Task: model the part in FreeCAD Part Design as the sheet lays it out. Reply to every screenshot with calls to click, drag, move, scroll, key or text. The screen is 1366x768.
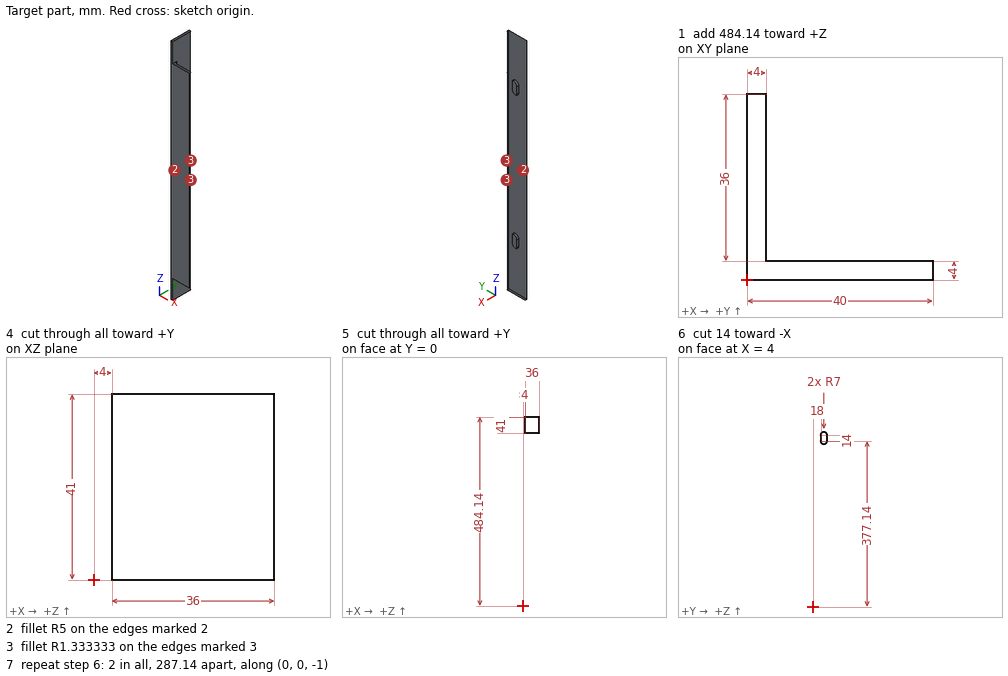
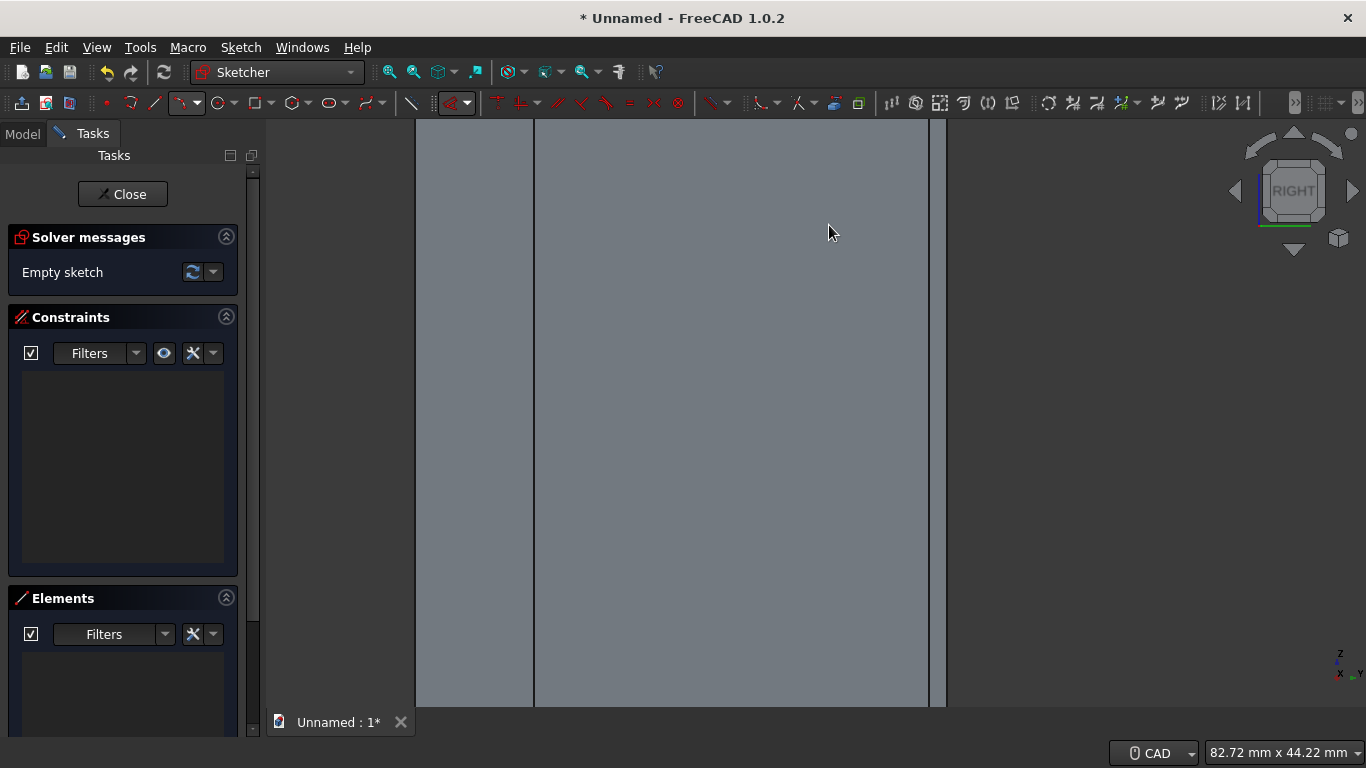
click(330, 104)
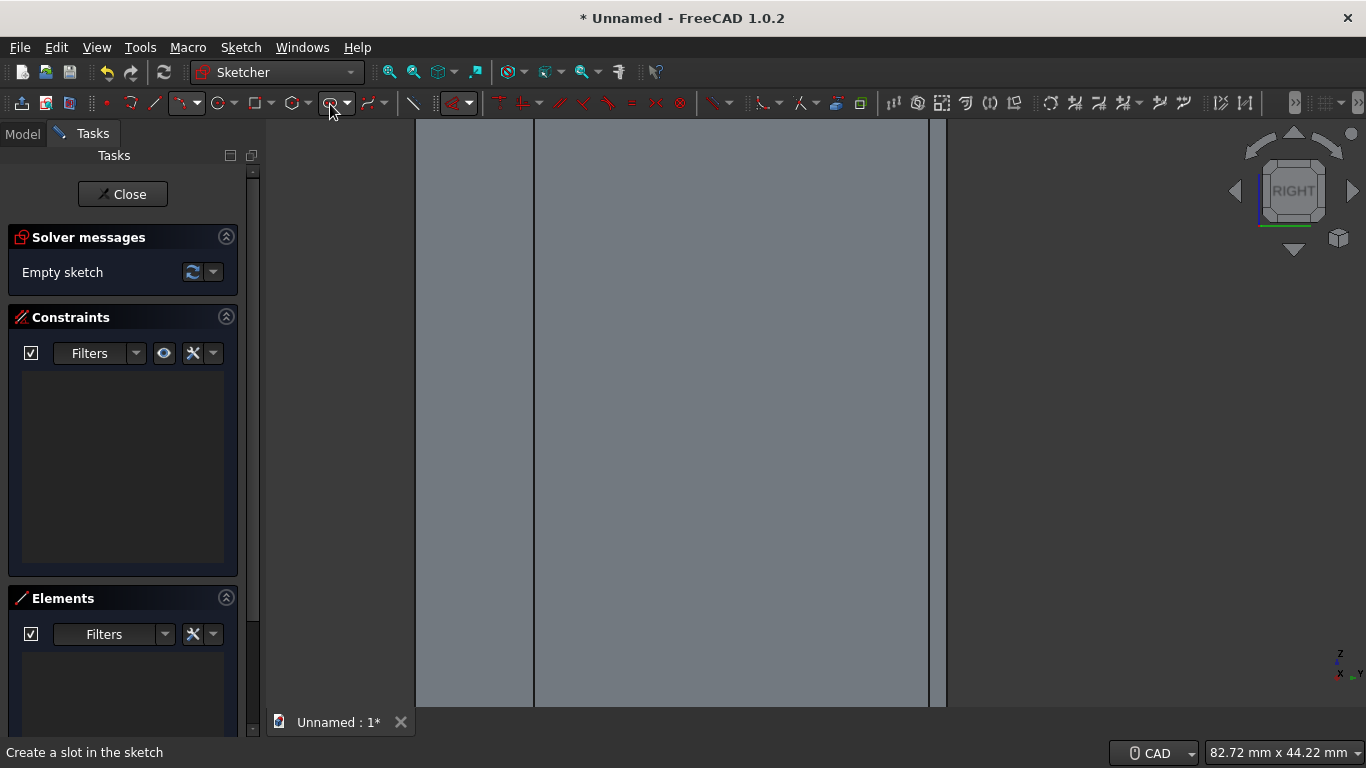
click(747, 499)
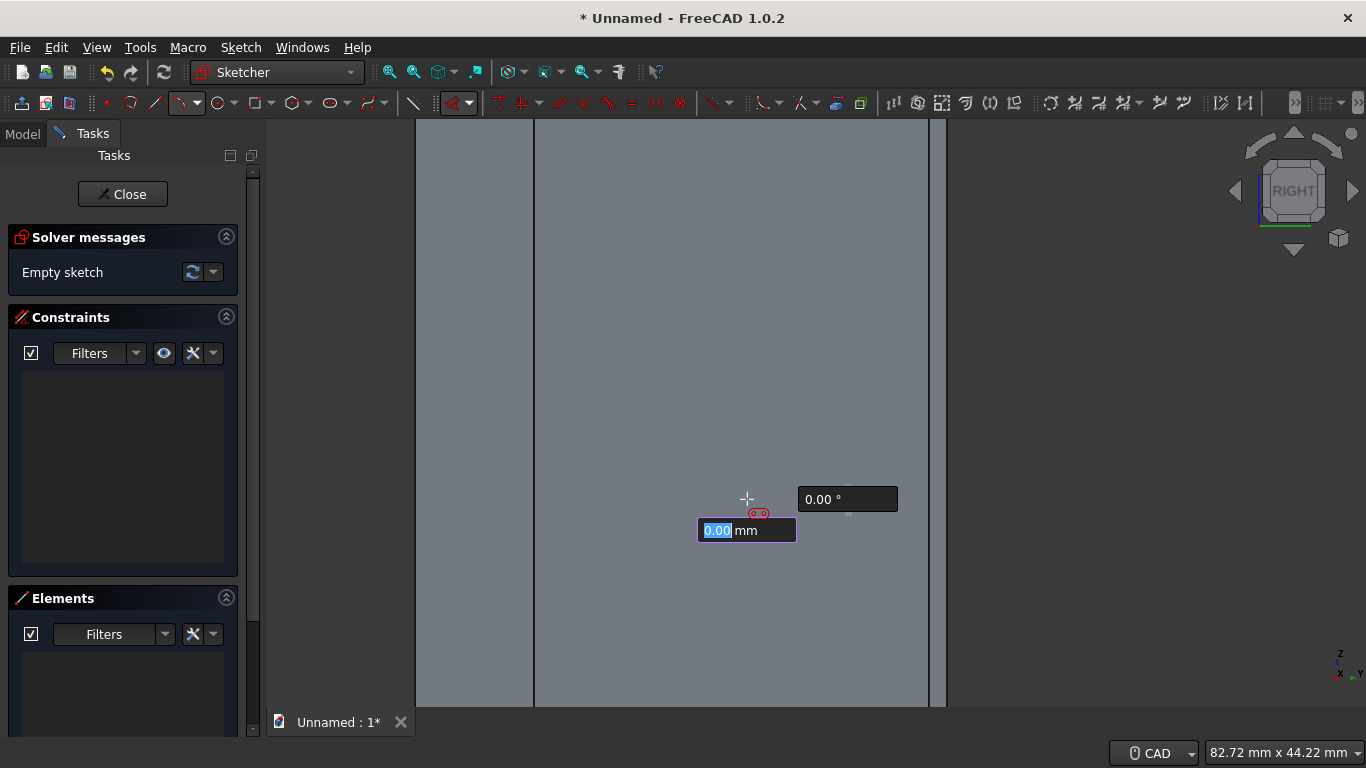
click(747, 313)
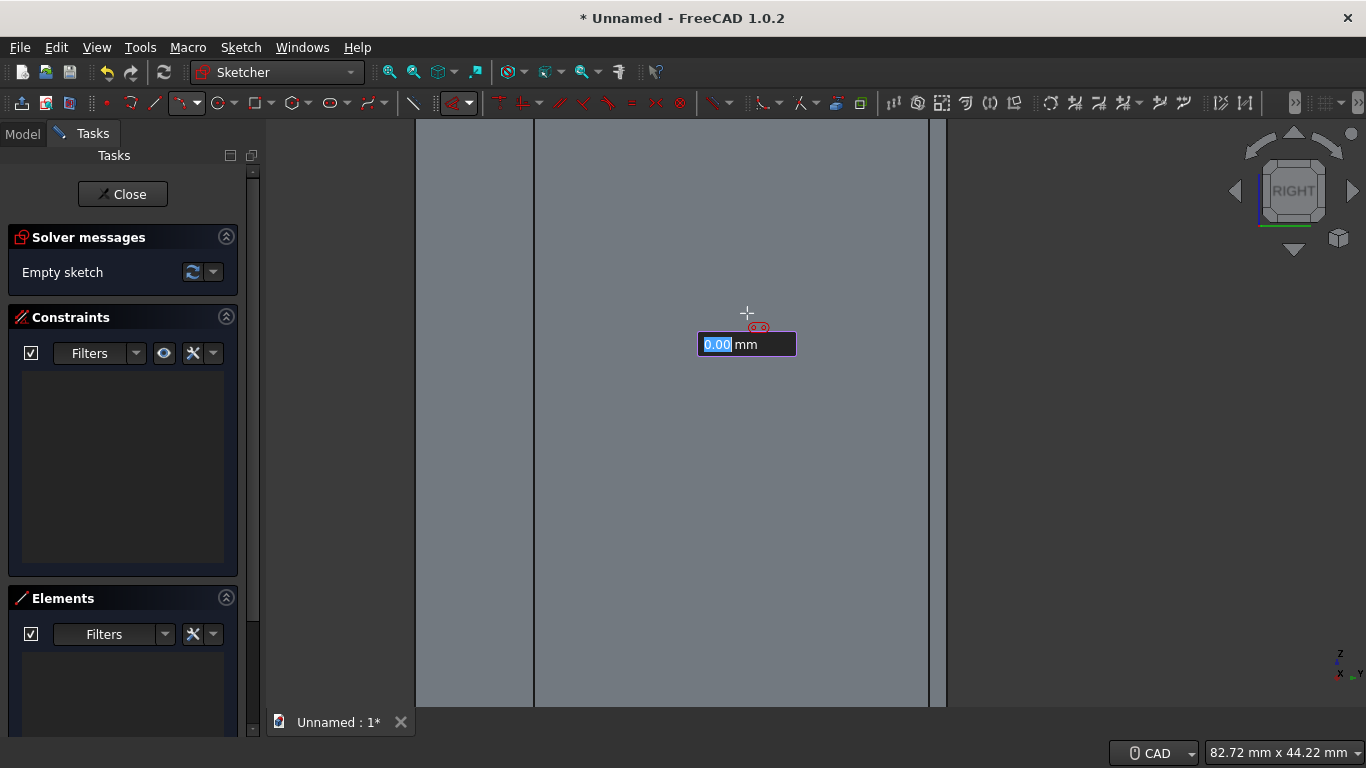
click(840, 406)
key(Escape)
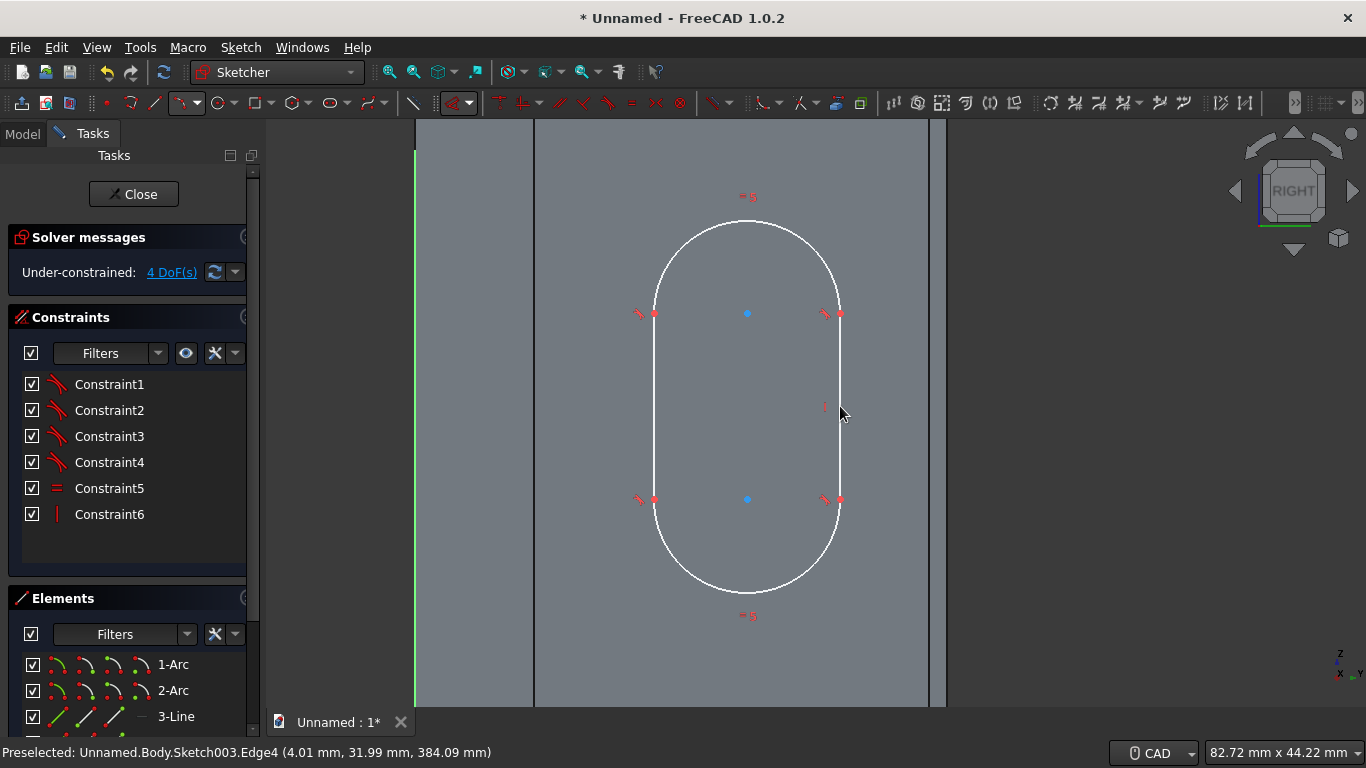
click(692, 575)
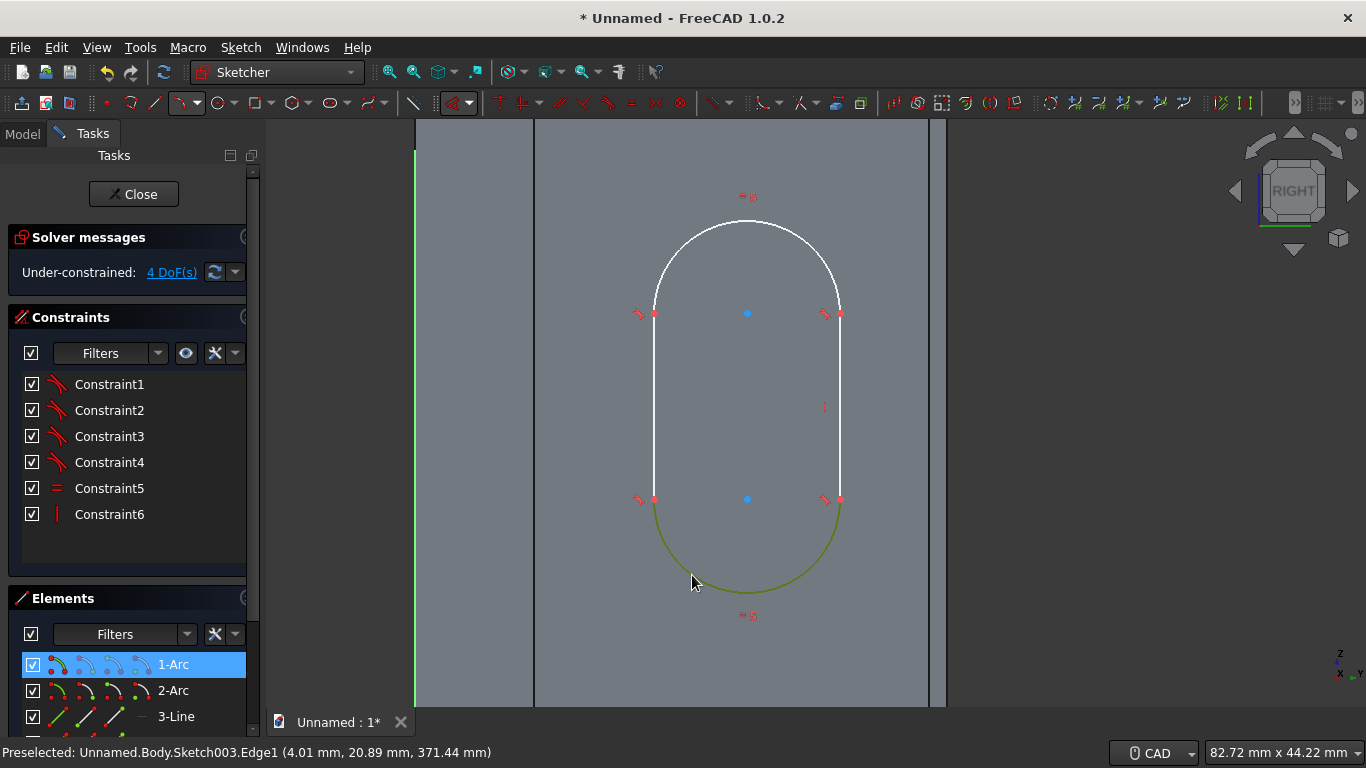
click(472, 104)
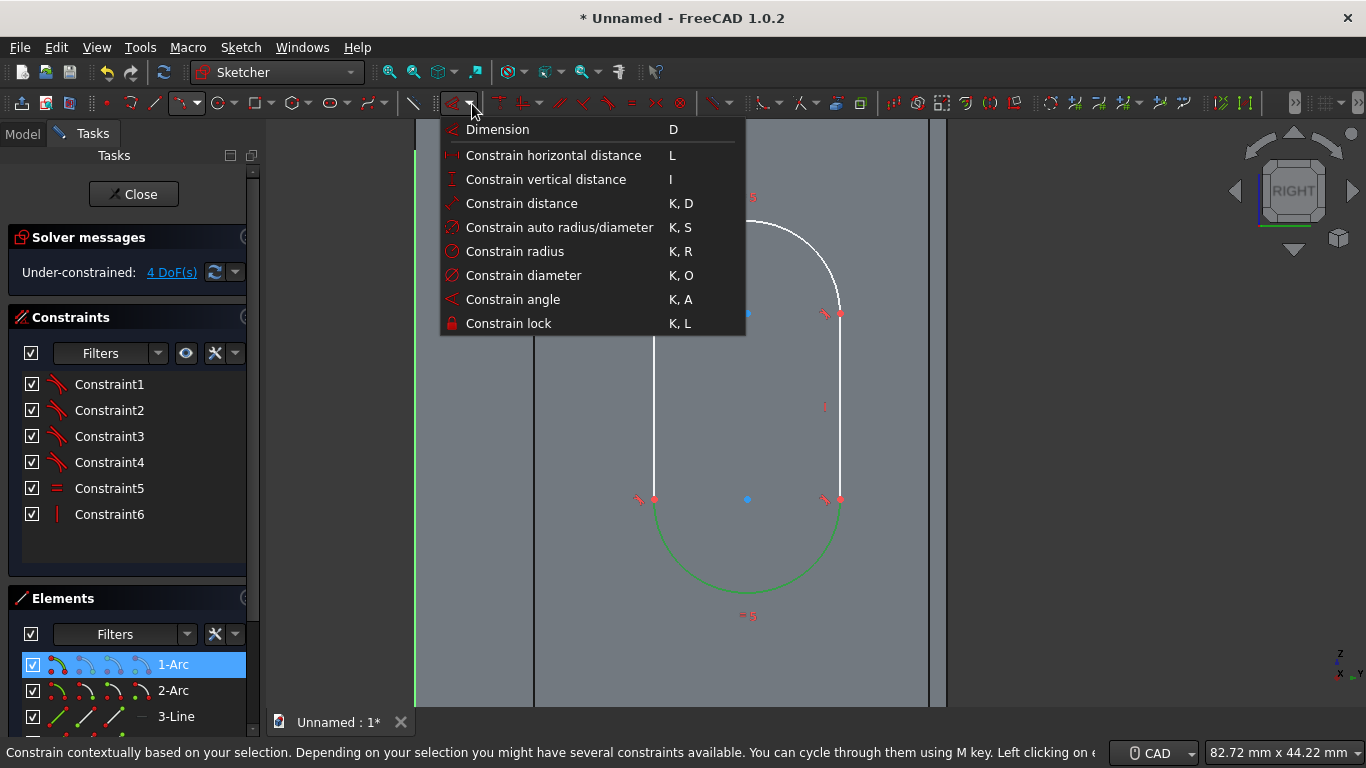
click(593, 251)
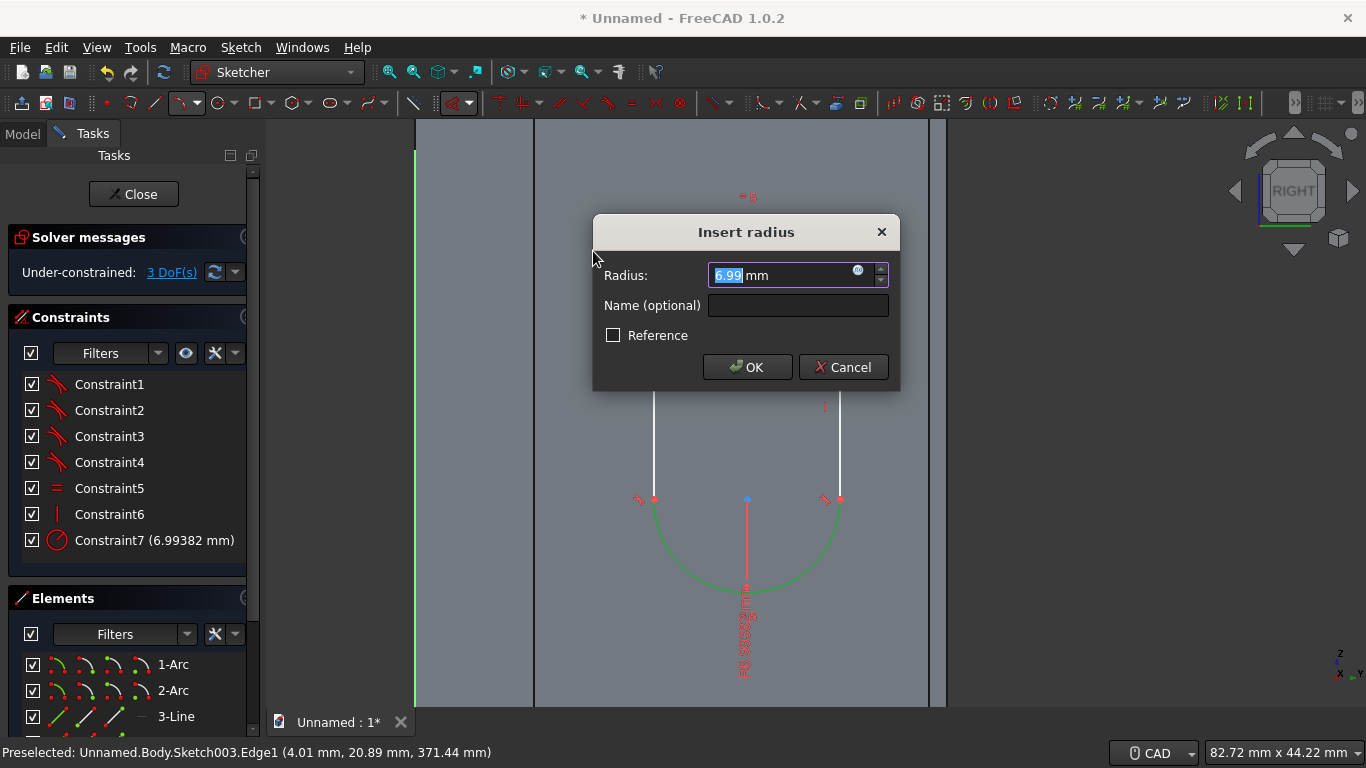
text(7)
key(Return)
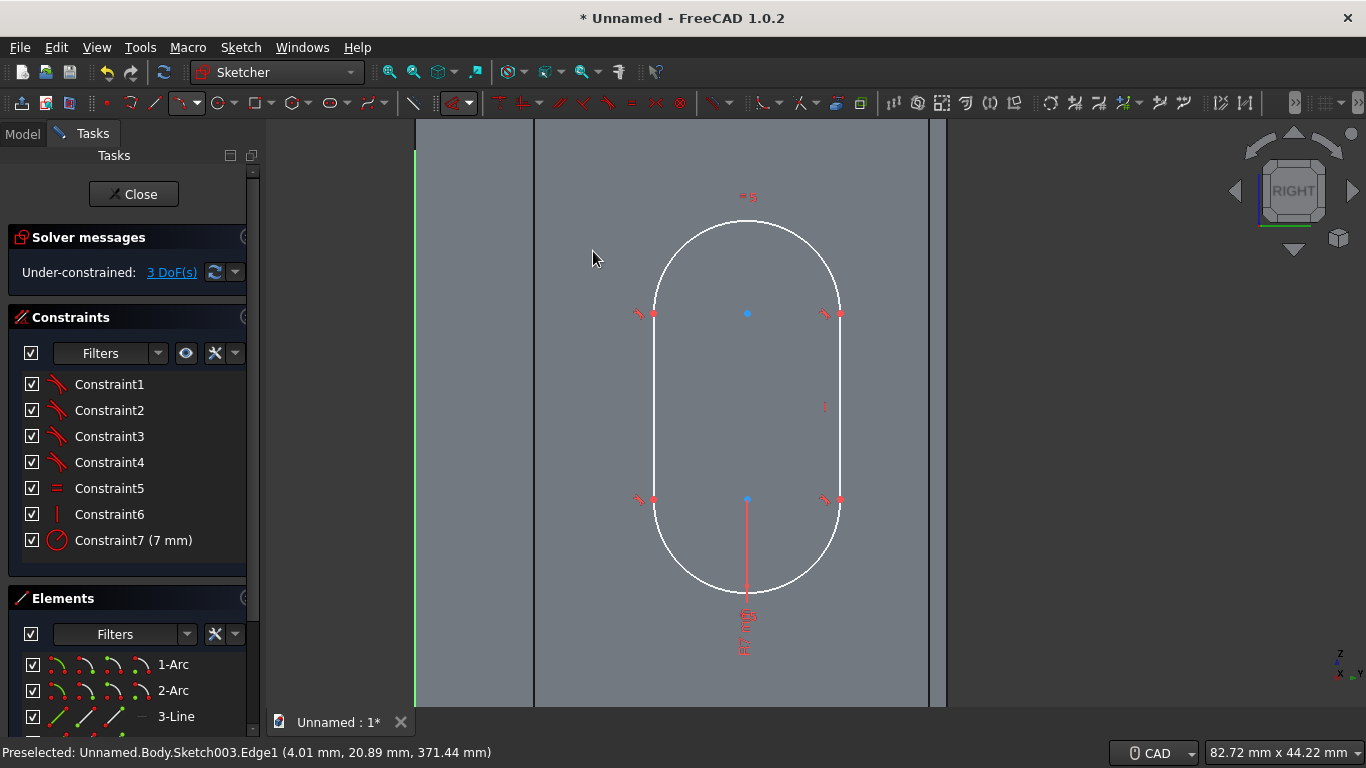
click(654, 444)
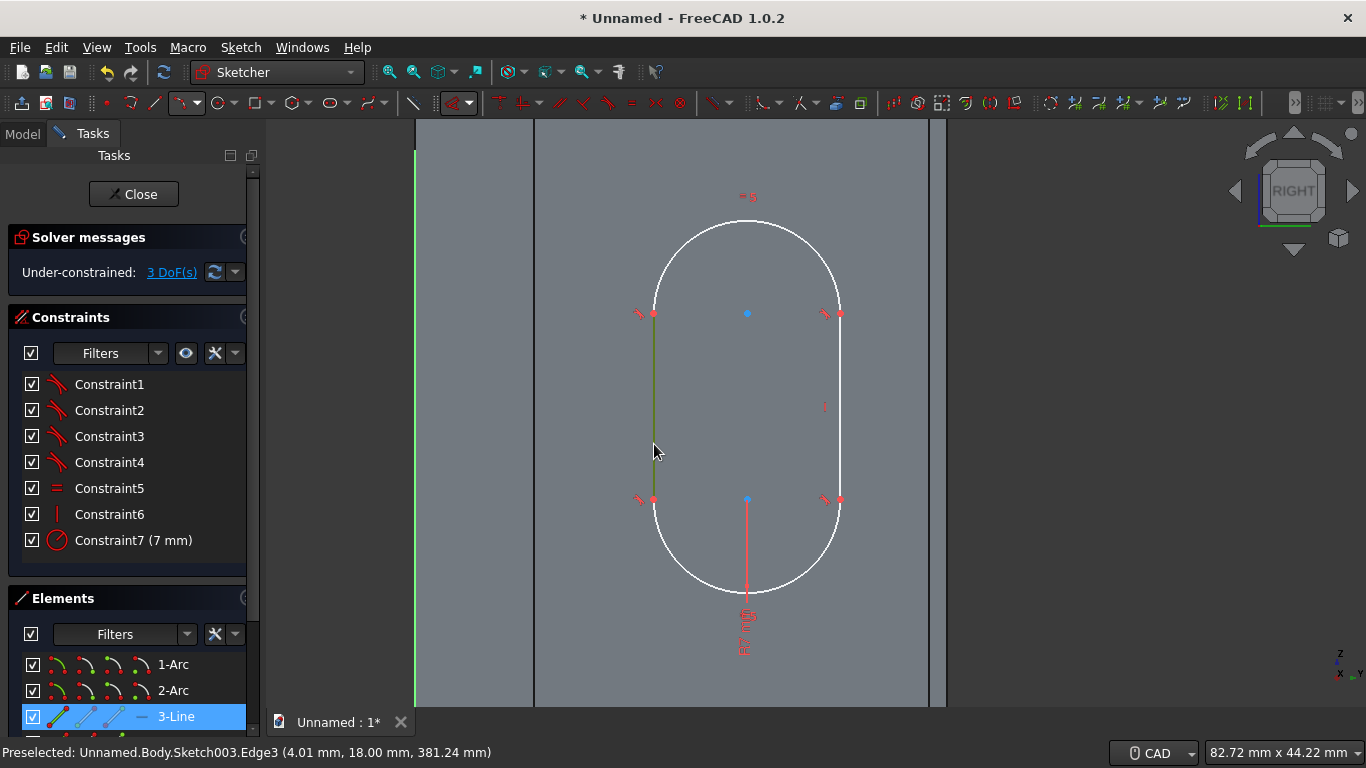
click(472, 104)